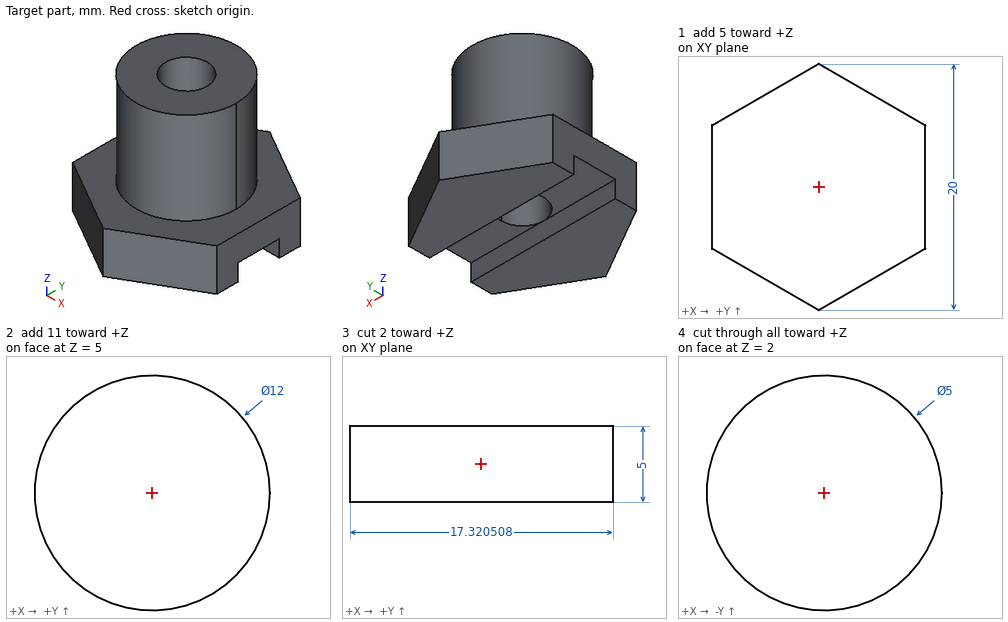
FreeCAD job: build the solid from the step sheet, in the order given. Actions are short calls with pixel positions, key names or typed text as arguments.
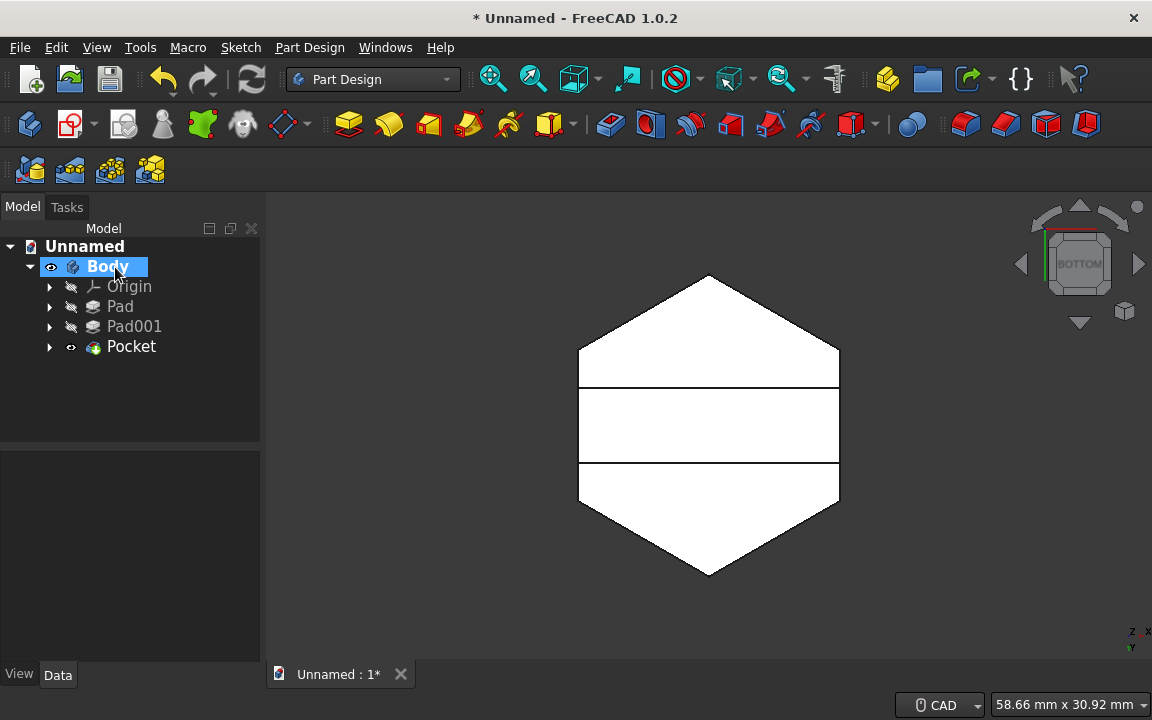
click(784, 424)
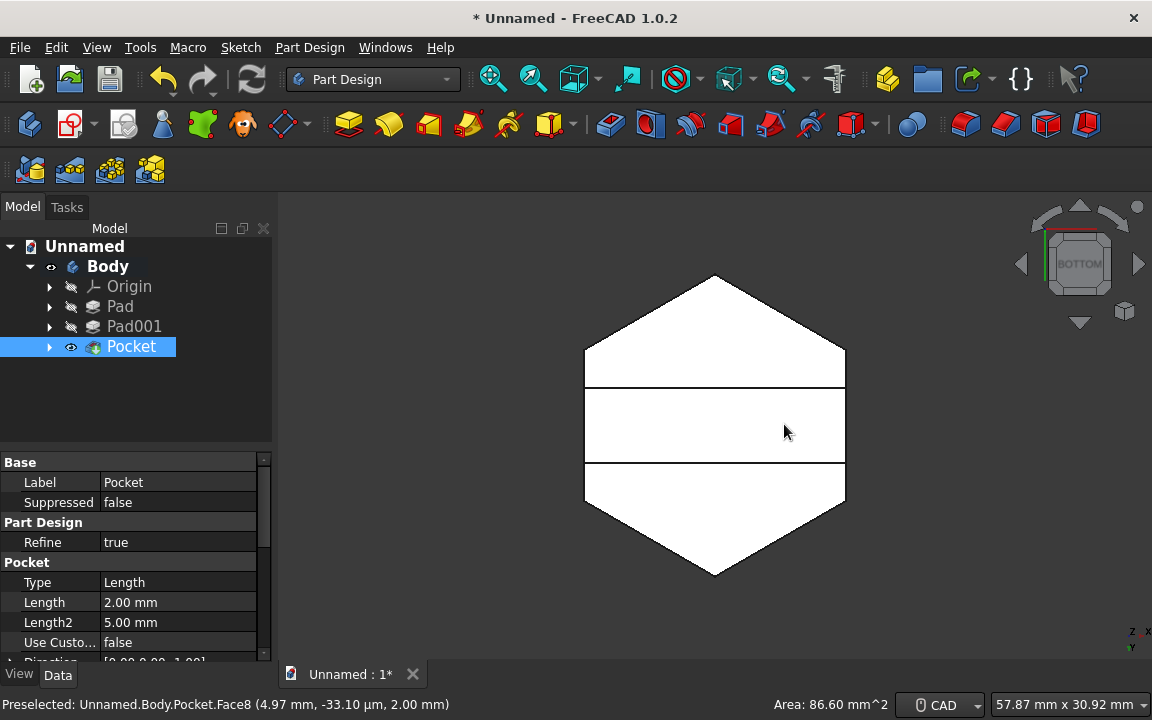
click(70, 124)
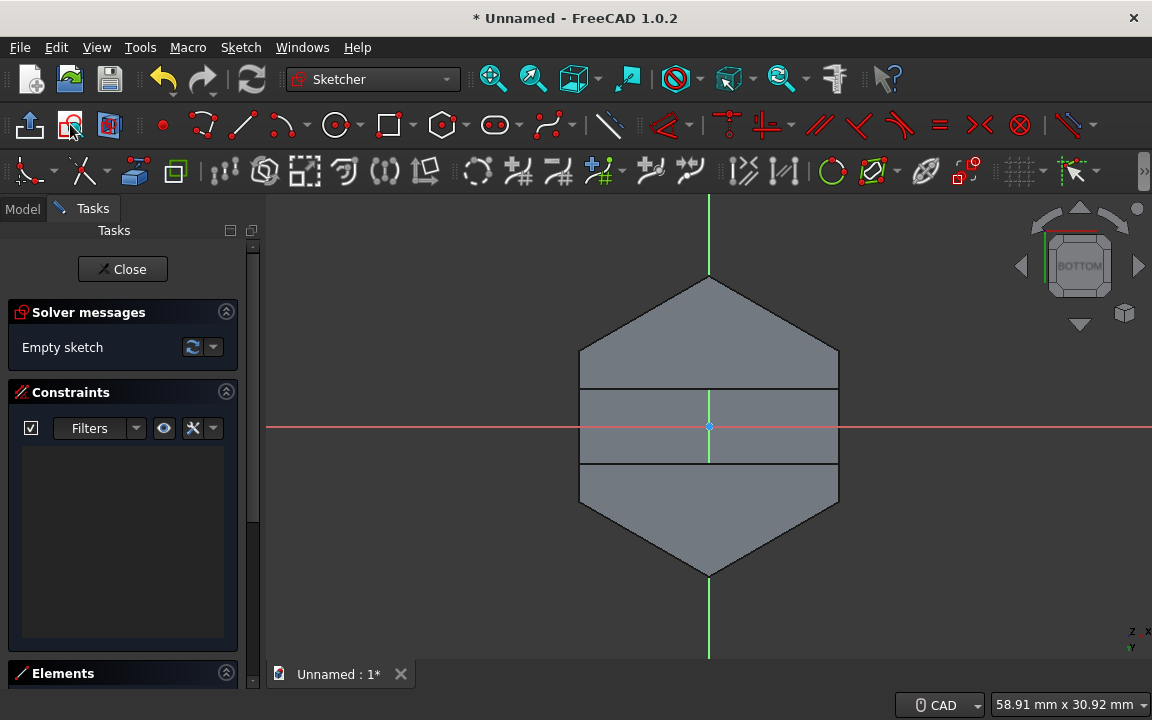
scroll(731, 426, up, 7)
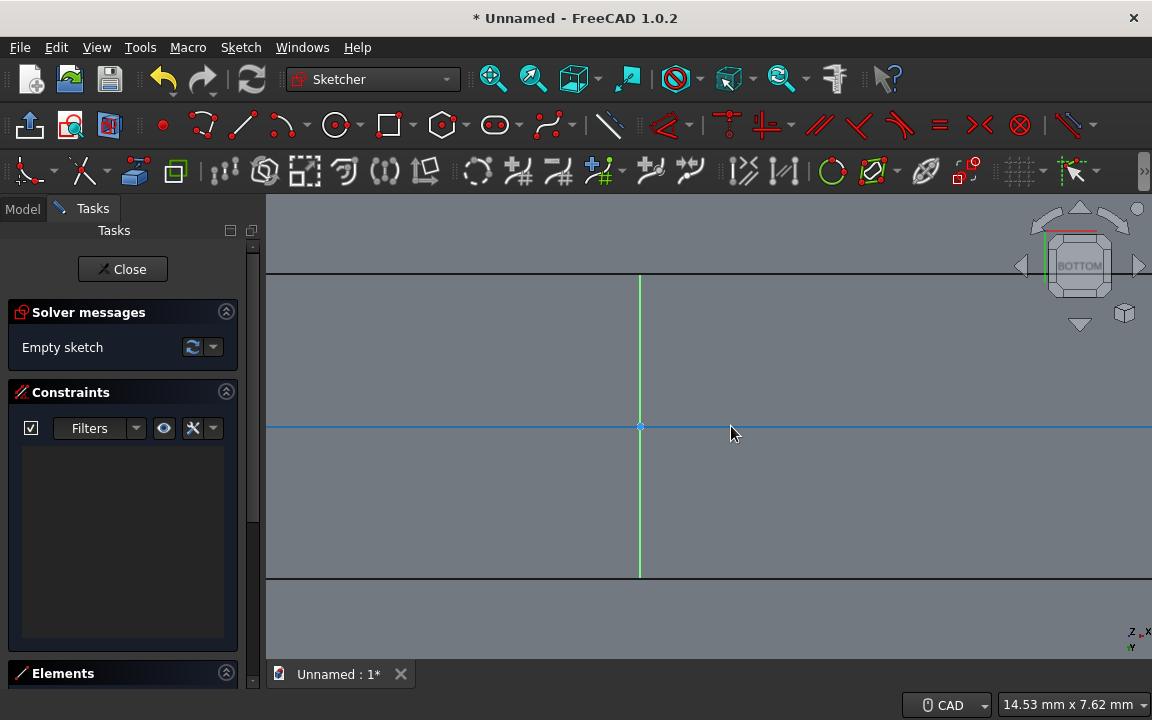
key(g)
key(c)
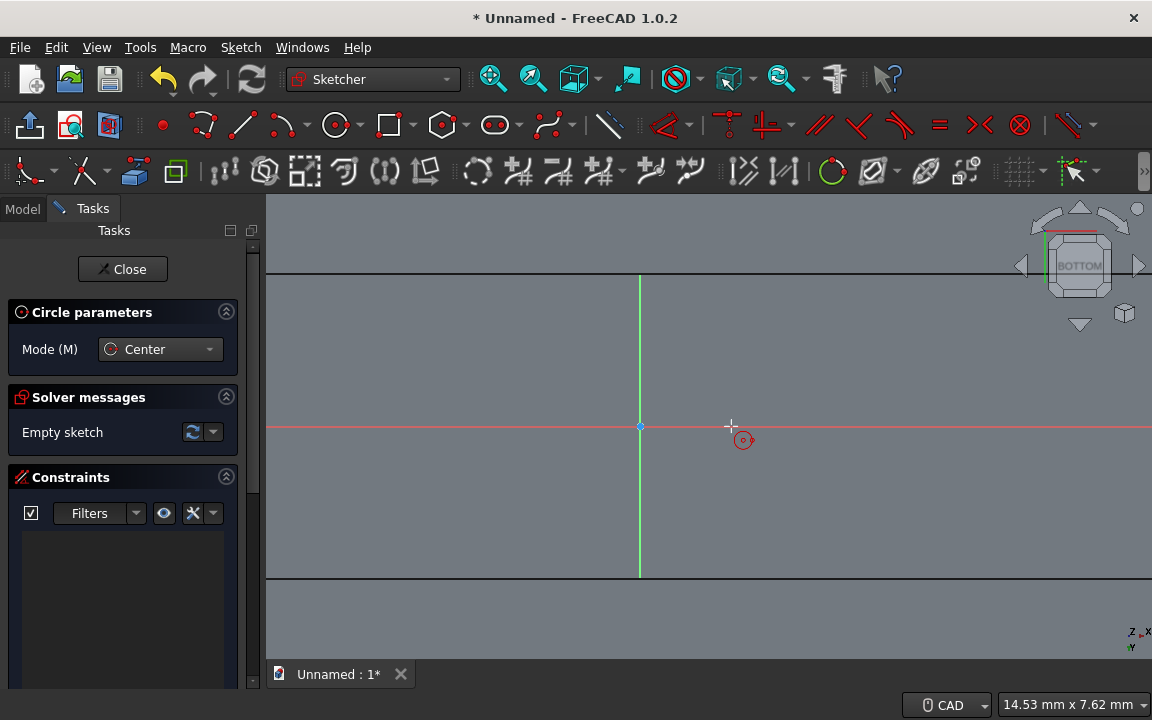
click(640, 426)
click(748, 319)
key(Escape)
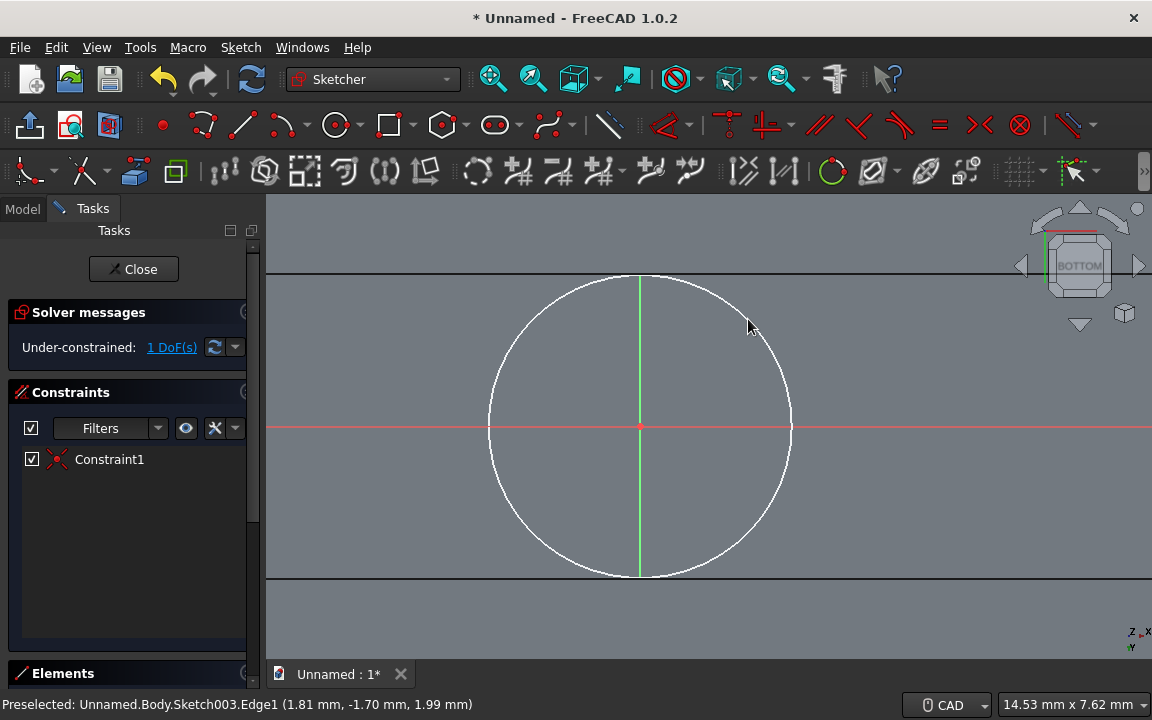
click(664, 126)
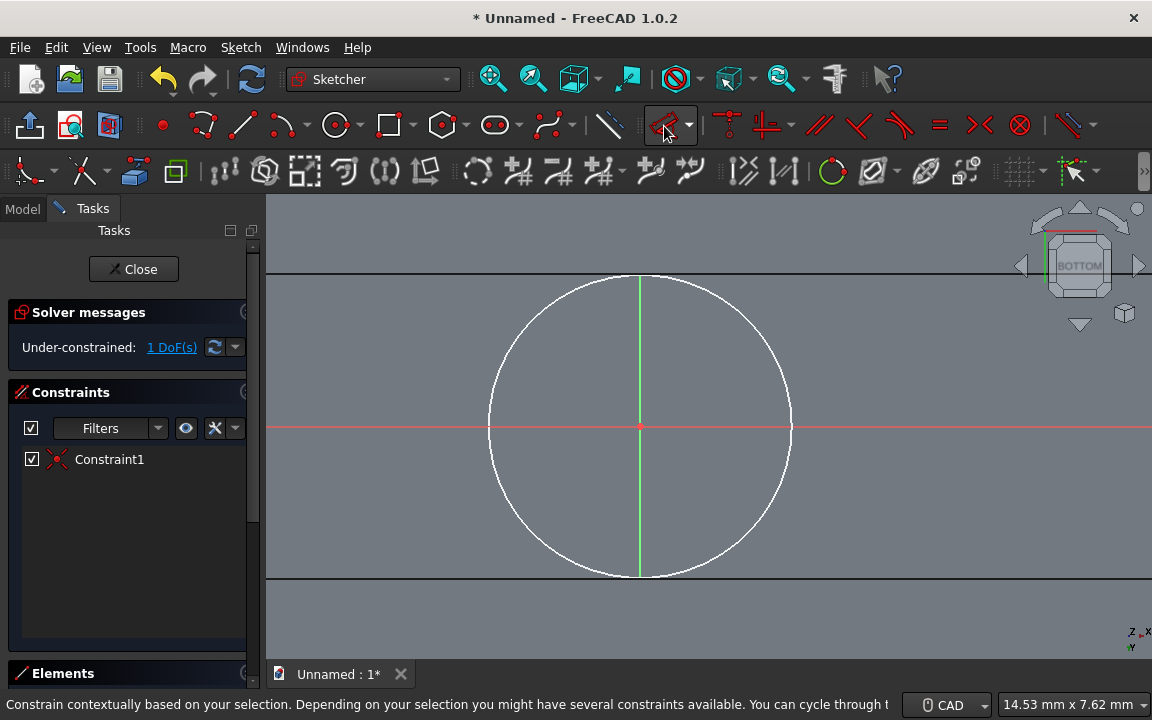
click(747, 319)
click(770, 296)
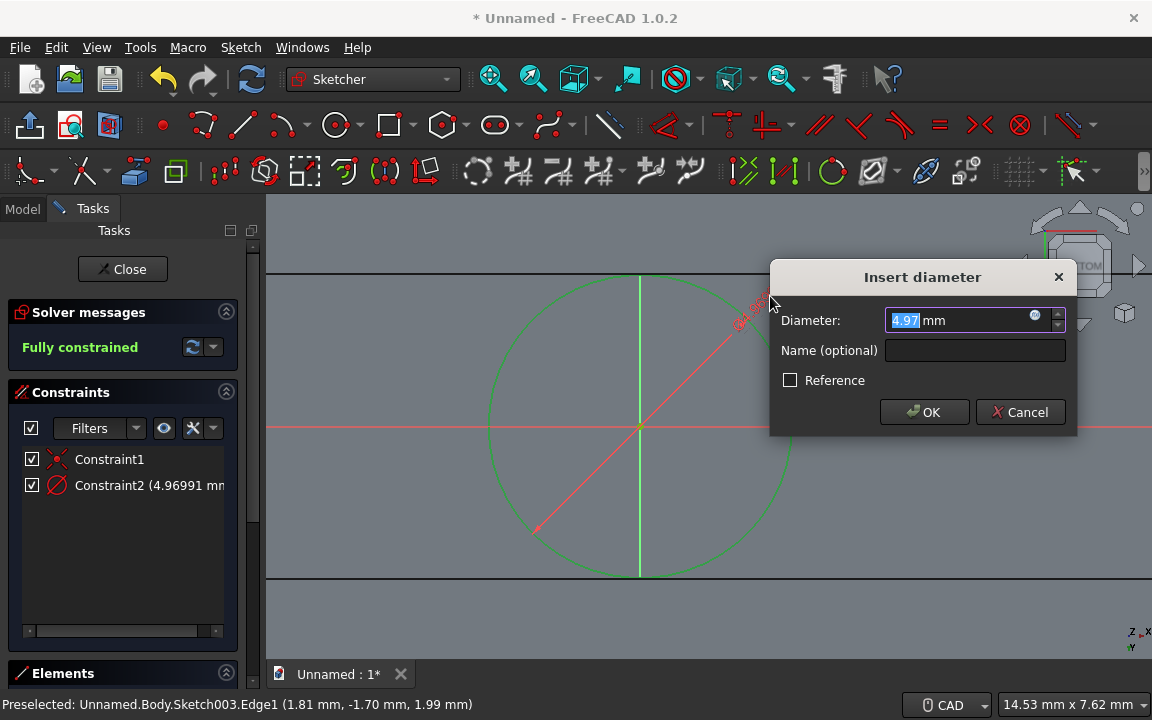
text(5)
key(Return)
key(Escape)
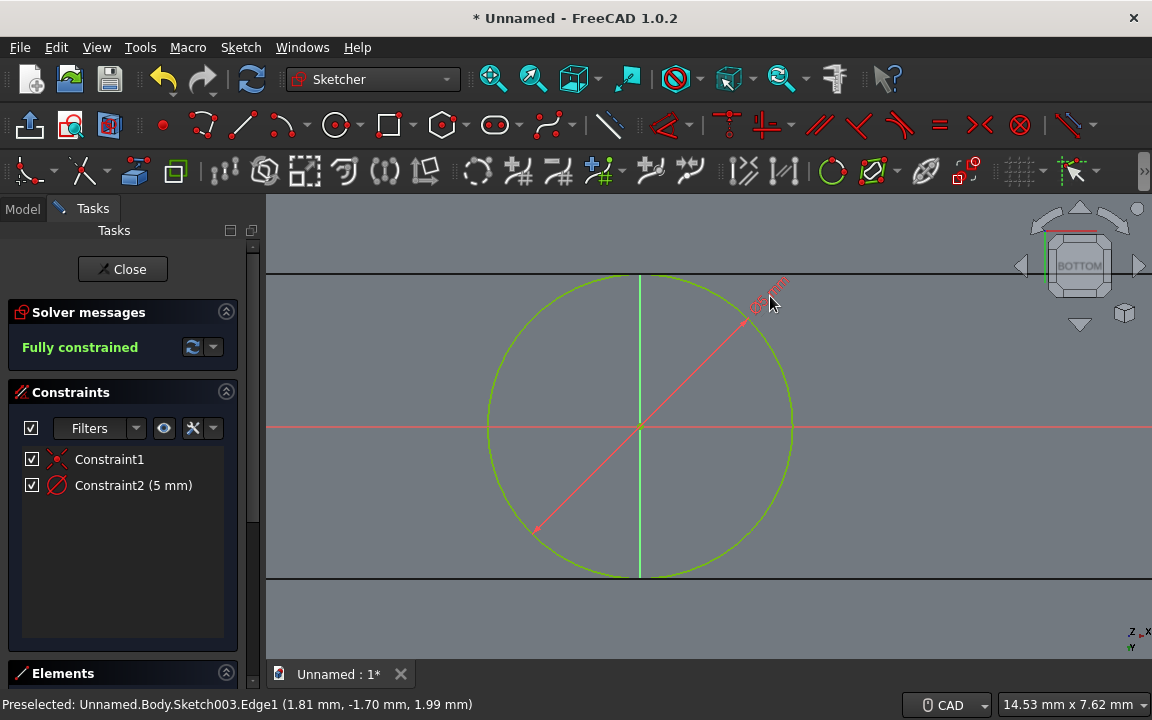
click(123, 269)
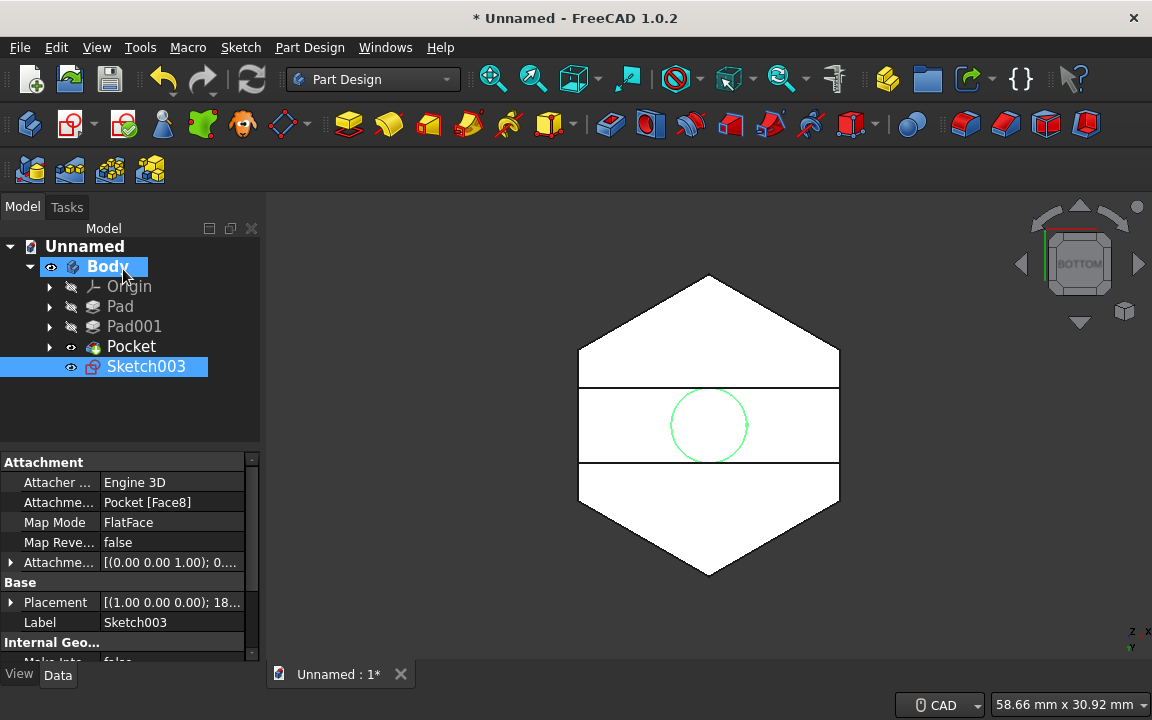
click(612, 124)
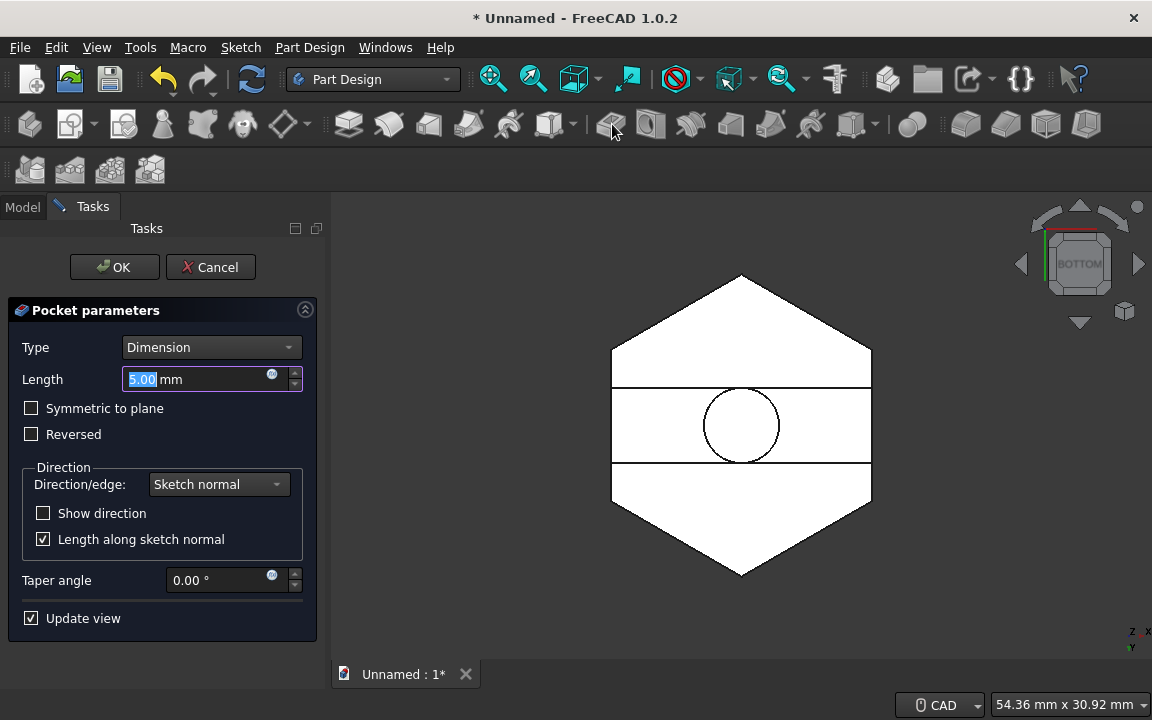
click(212, 348)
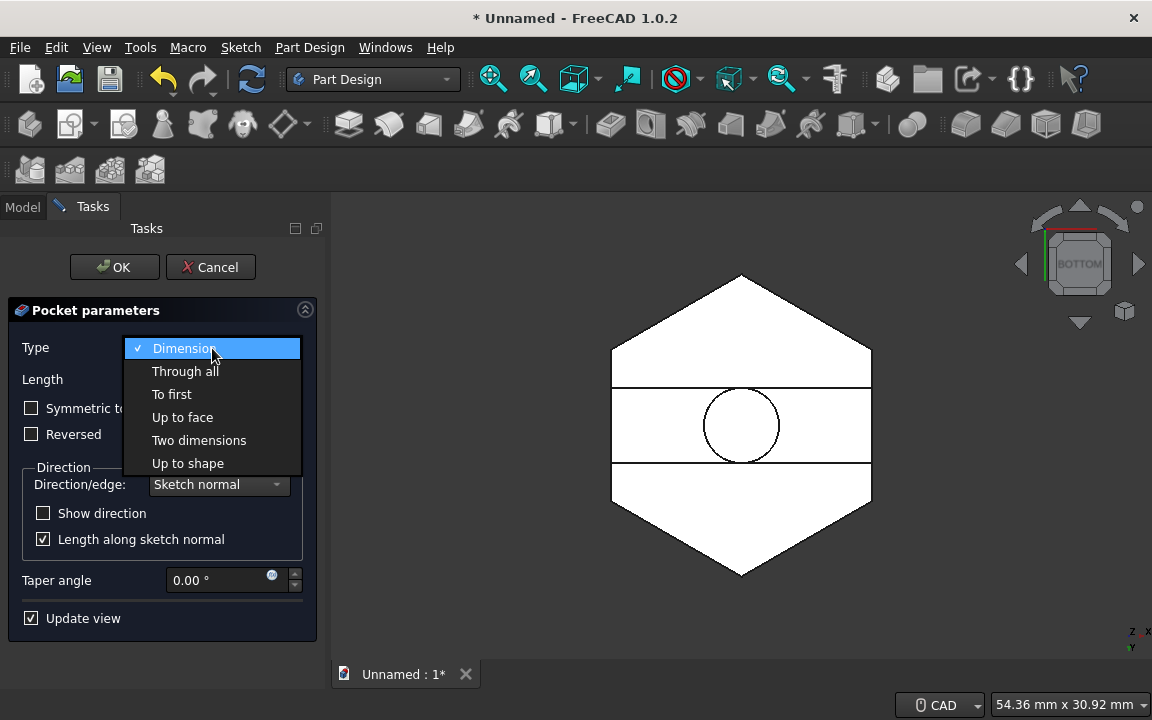
click(212, 372)